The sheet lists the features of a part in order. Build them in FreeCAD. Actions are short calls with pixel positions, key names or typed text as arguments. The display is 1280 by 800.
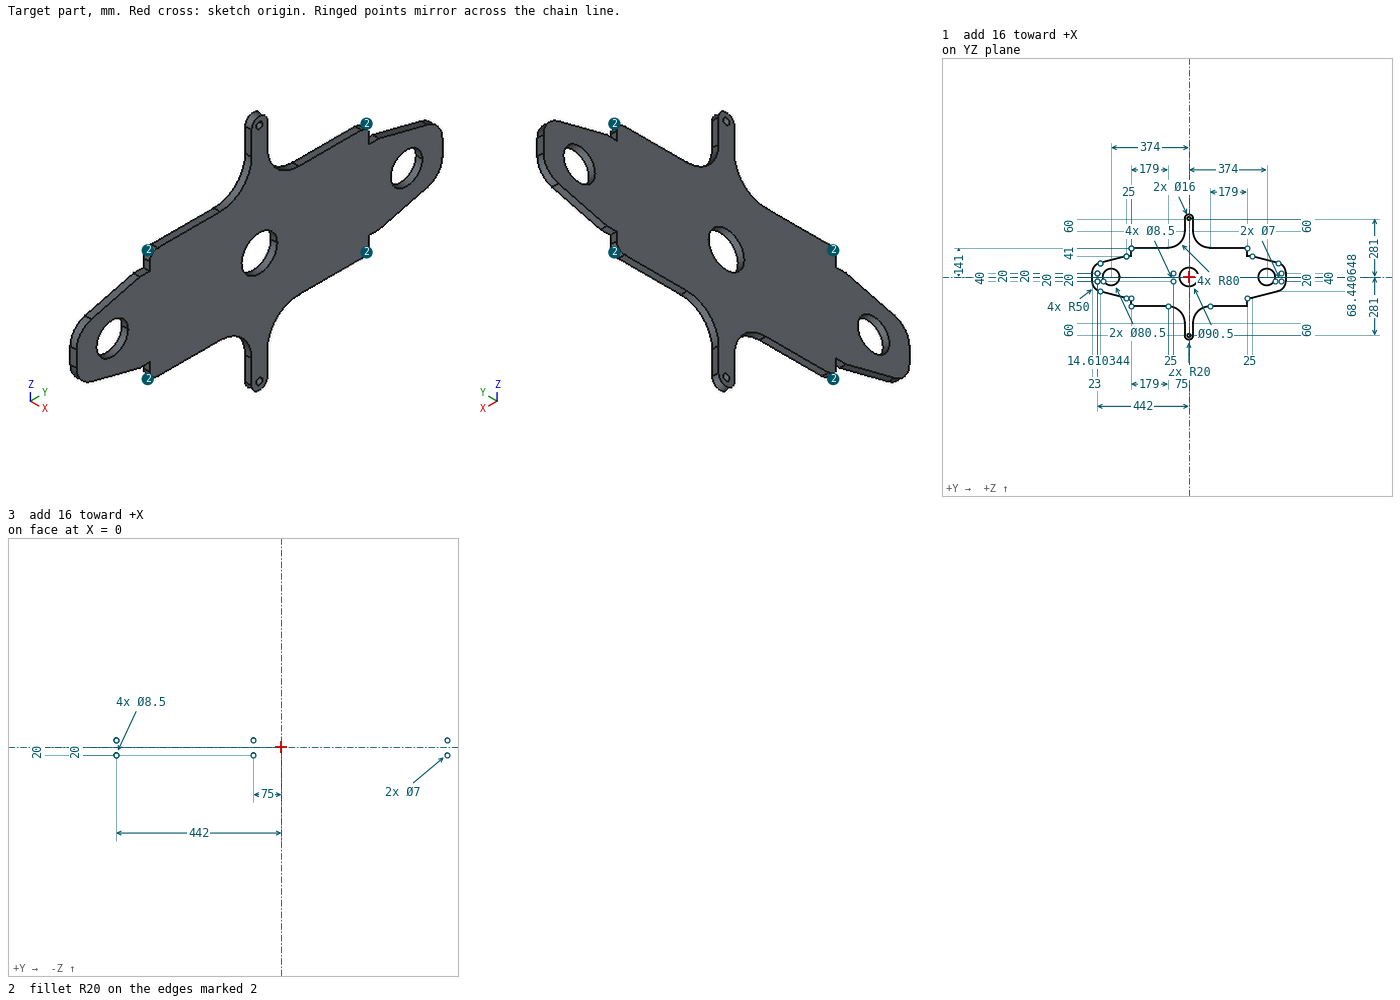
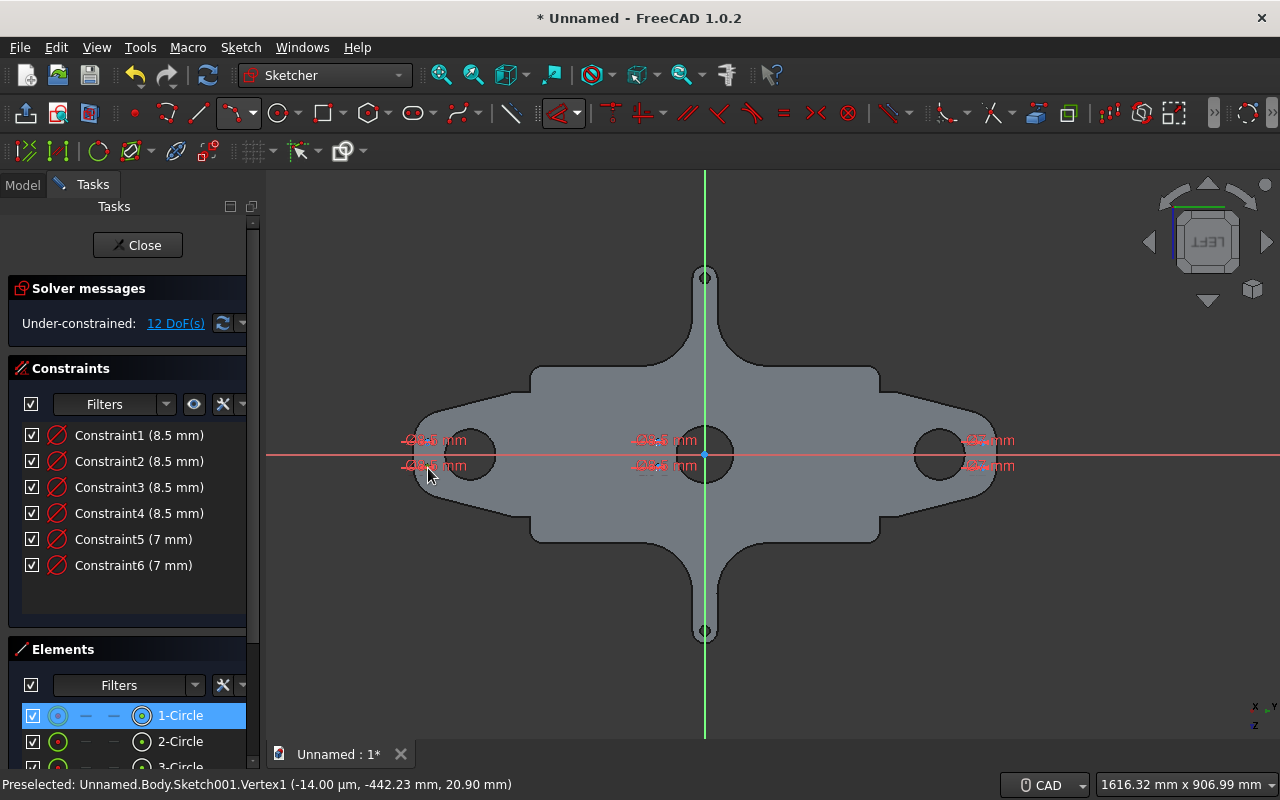
click(428, 442)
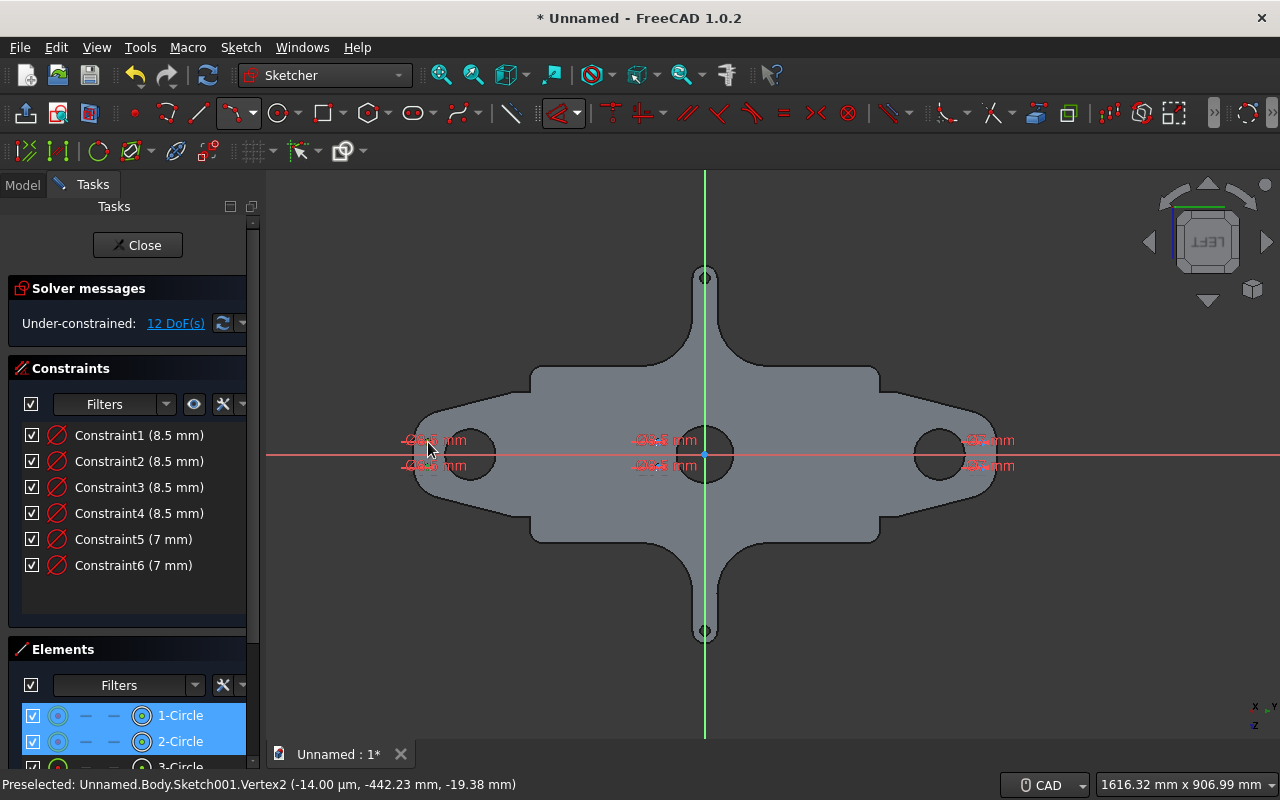
click(353, 455)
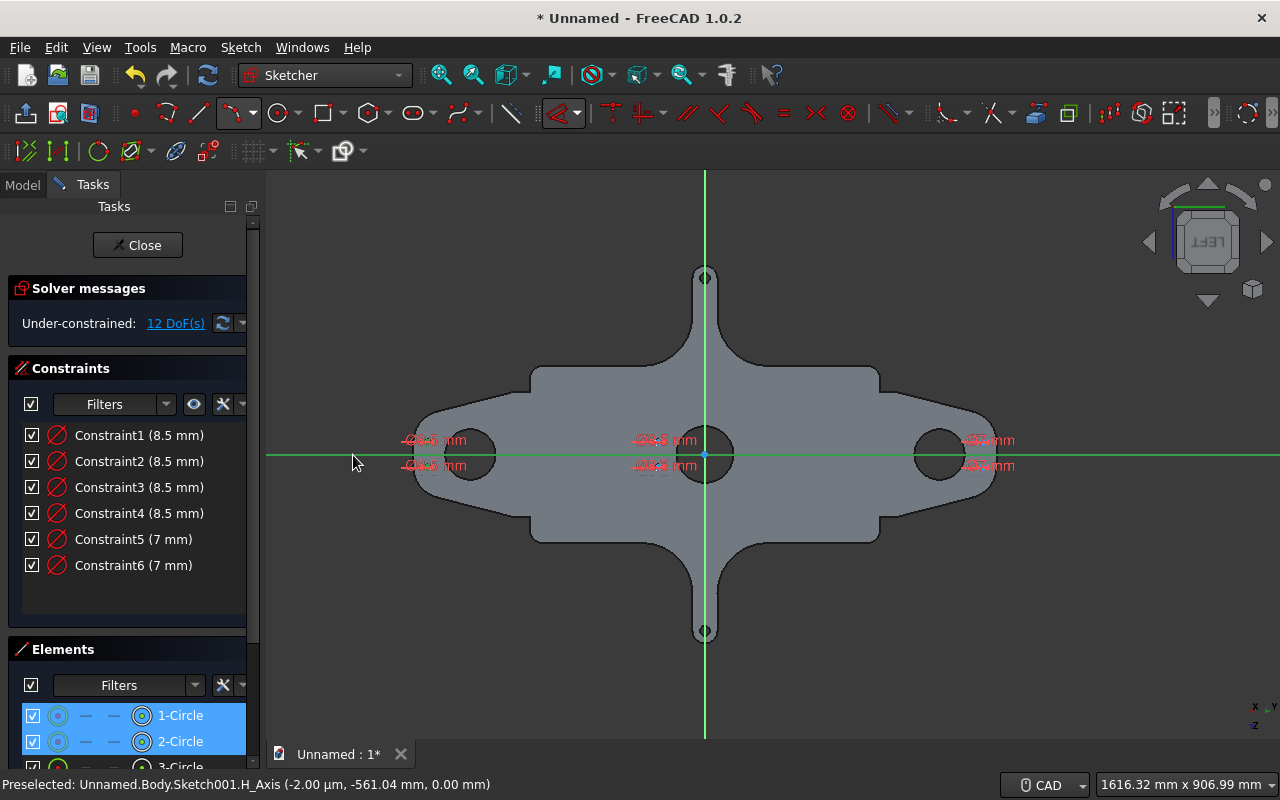
click(816, 114)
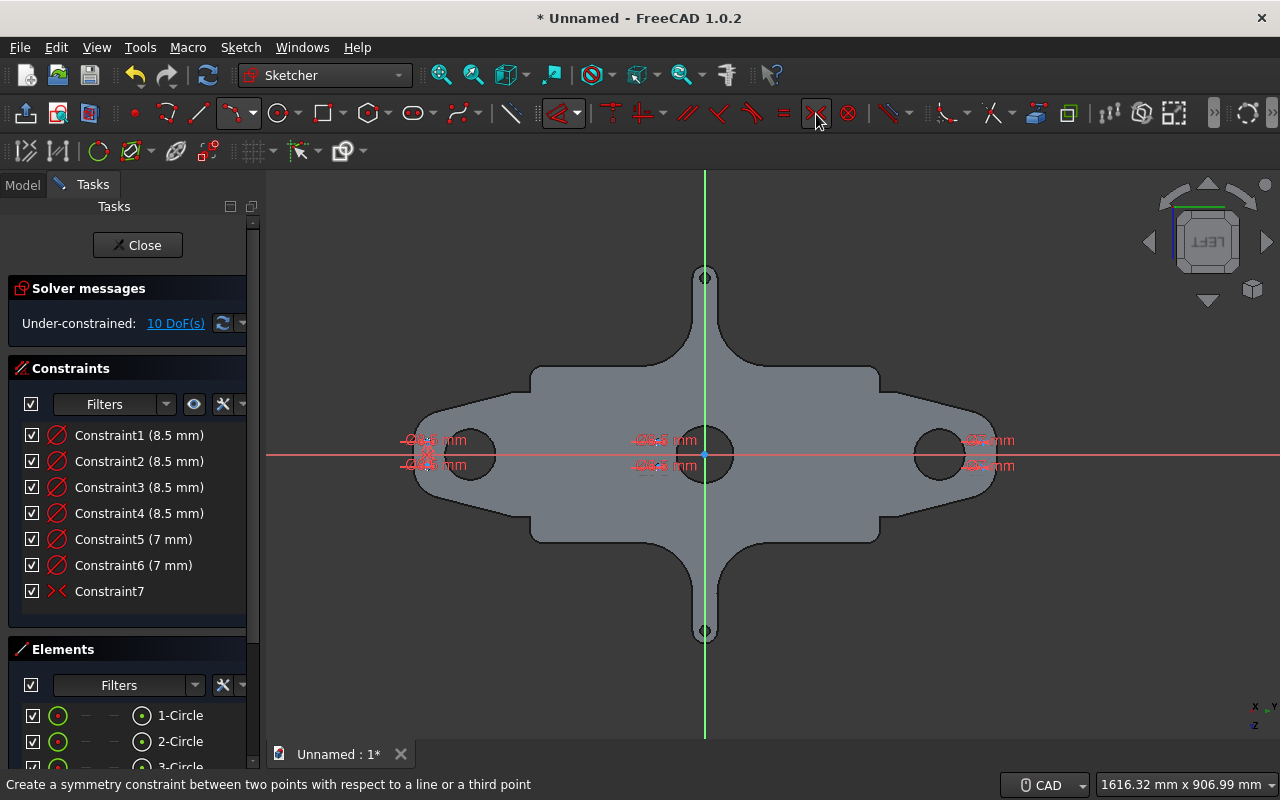
click(658, 468)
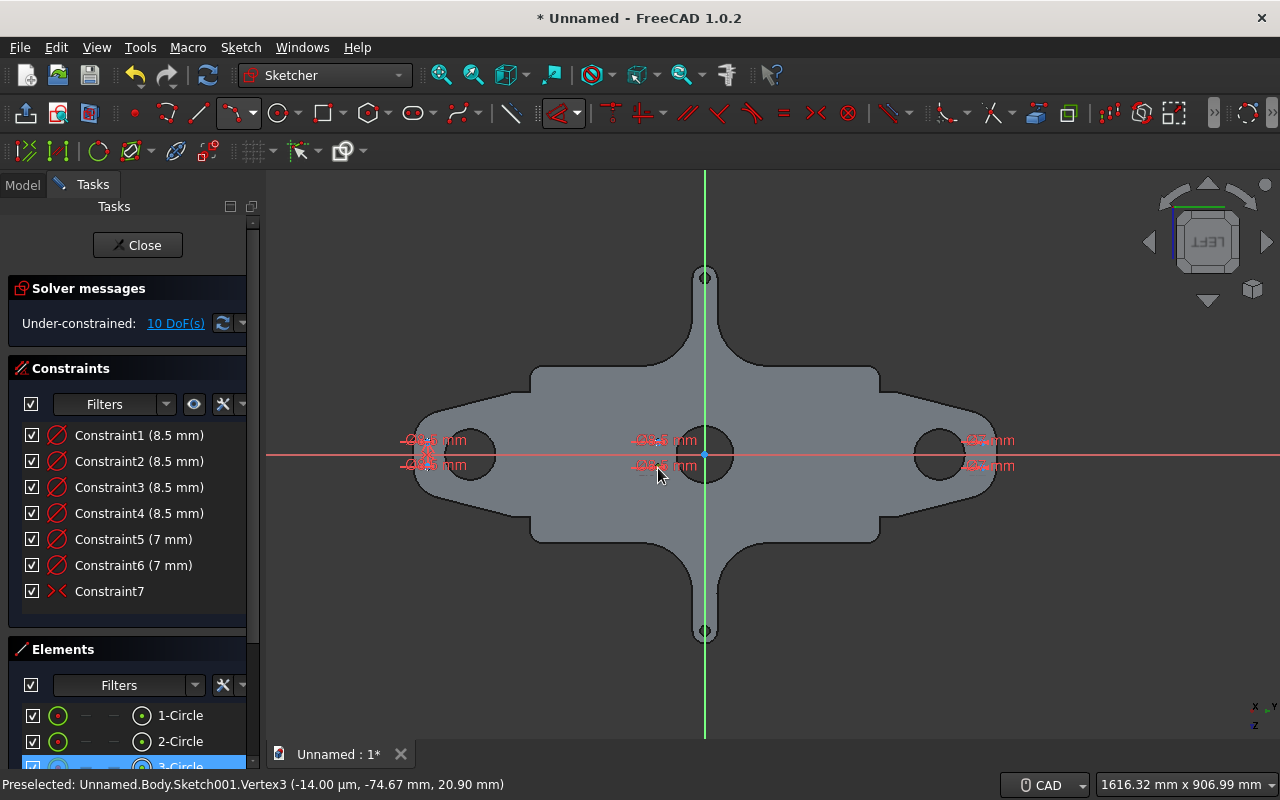
click(658, 442)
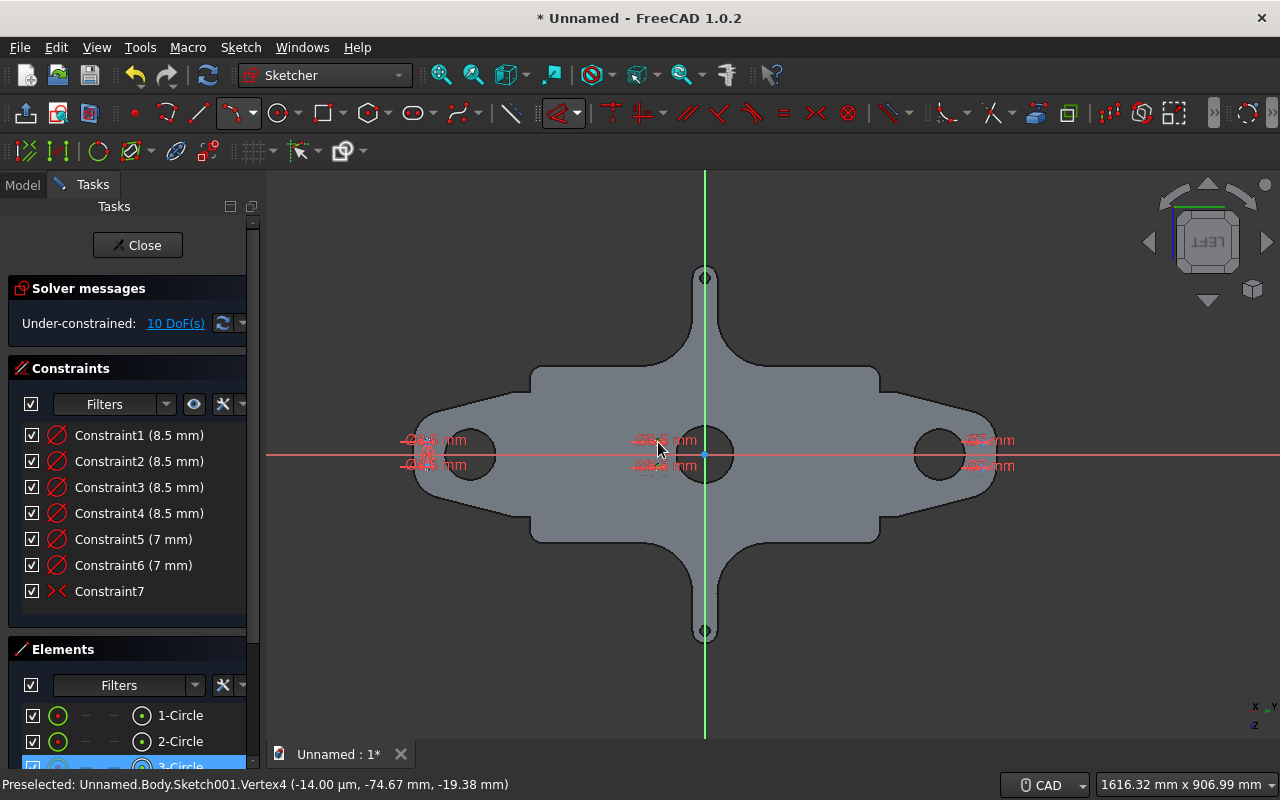
click(353, 455)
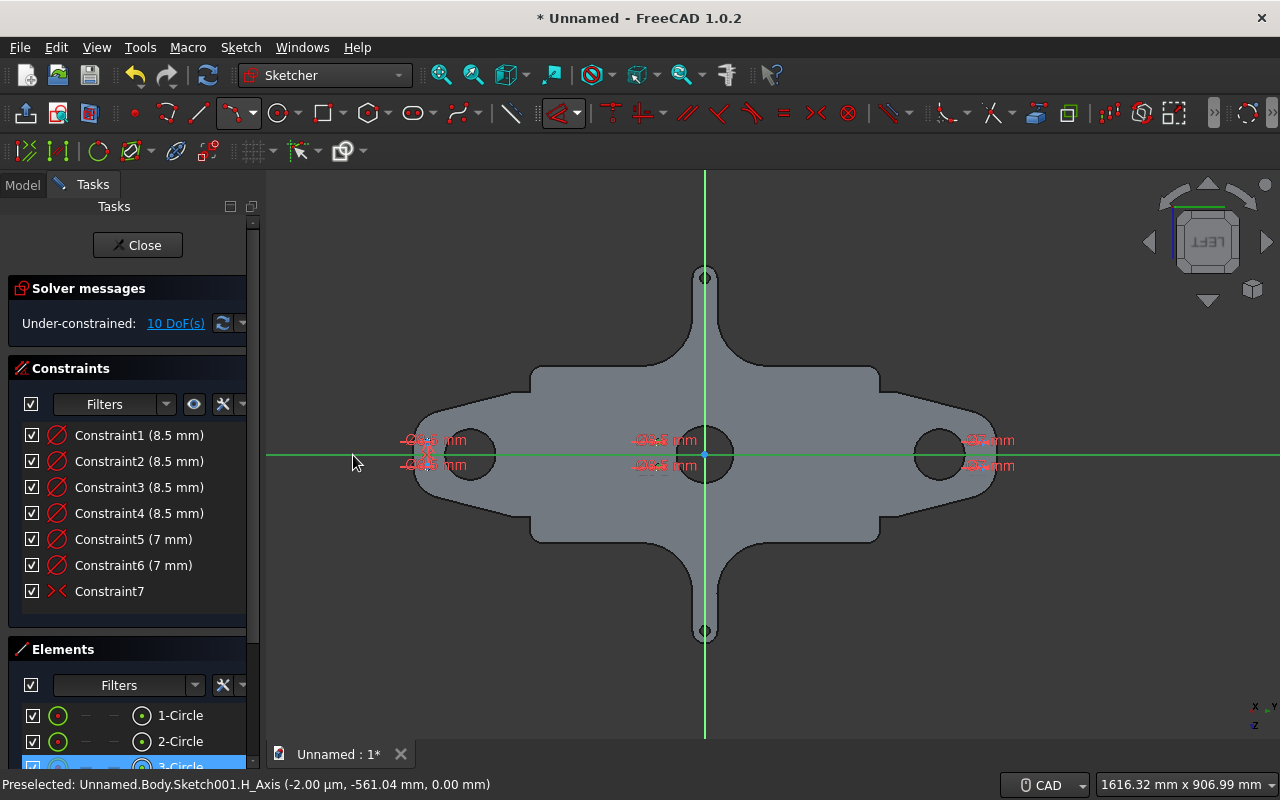
click(816, 114)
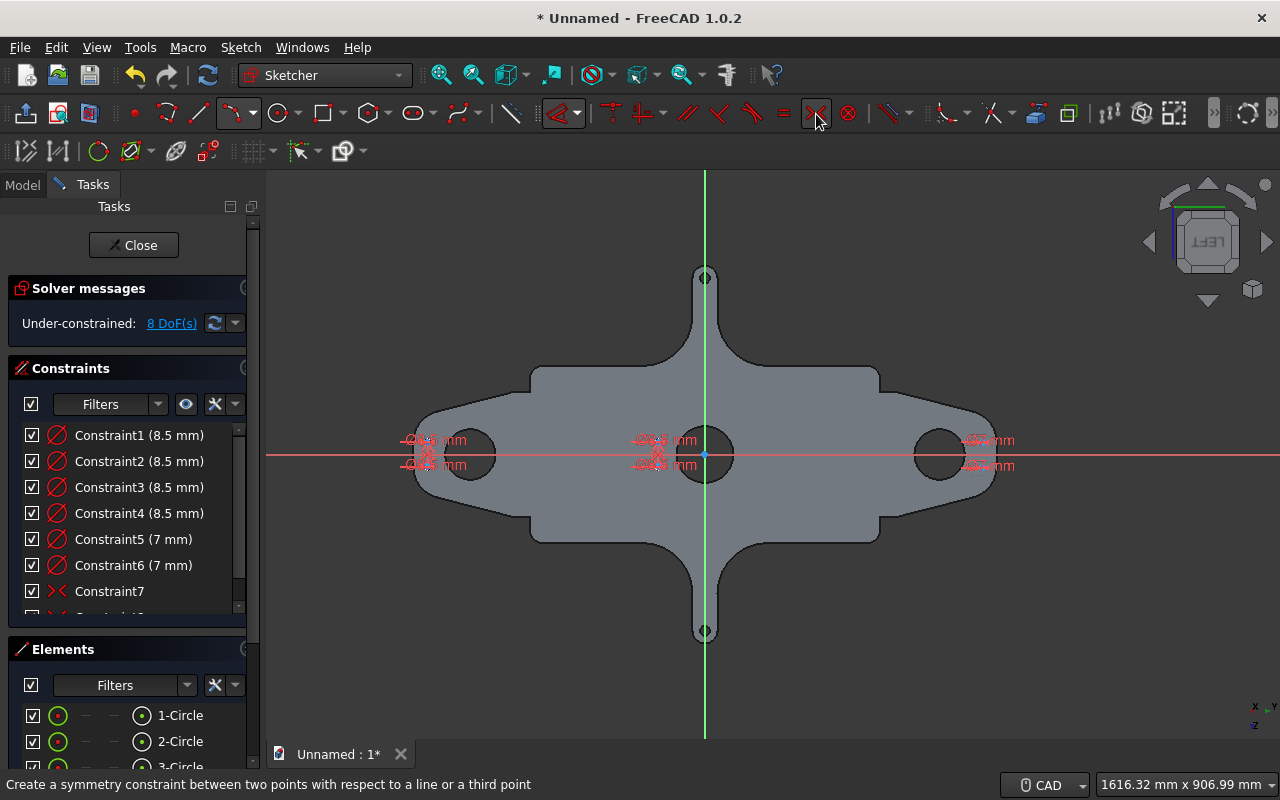
click(428, 467)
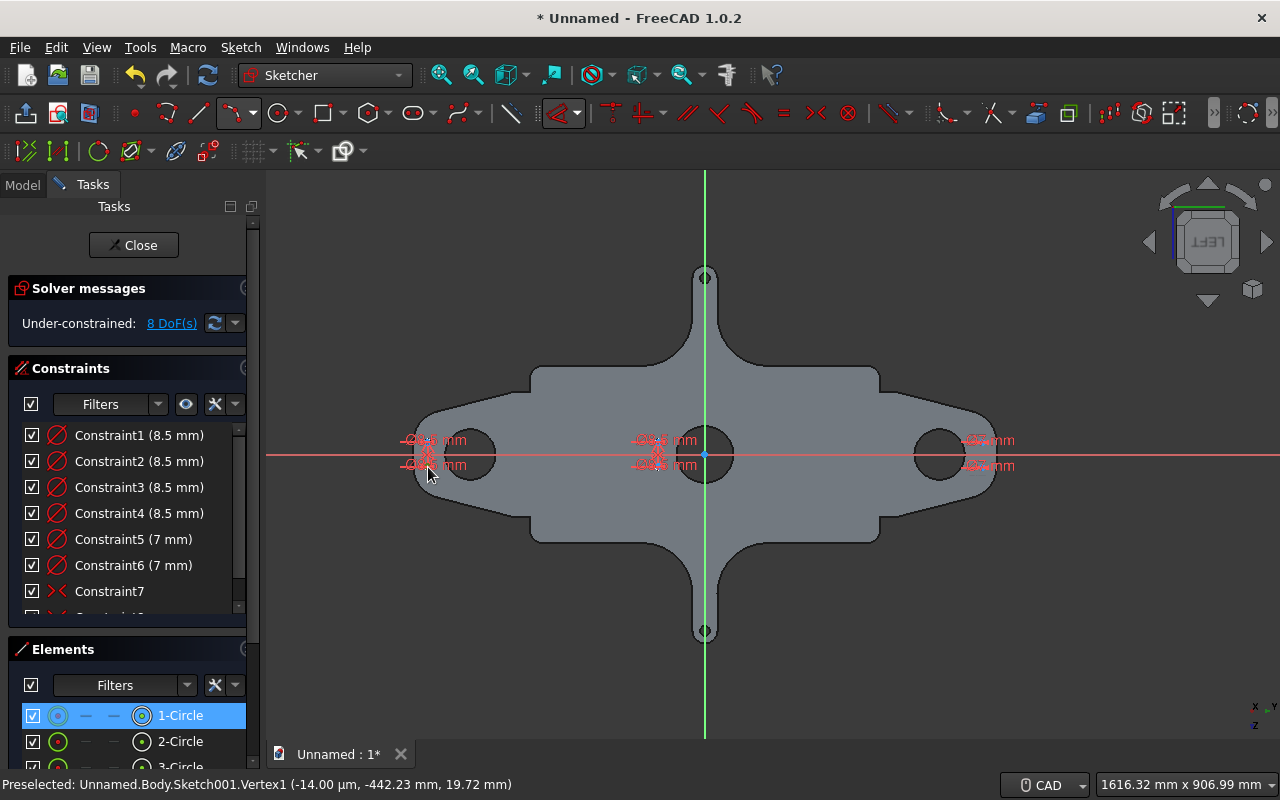
click(982, 468)